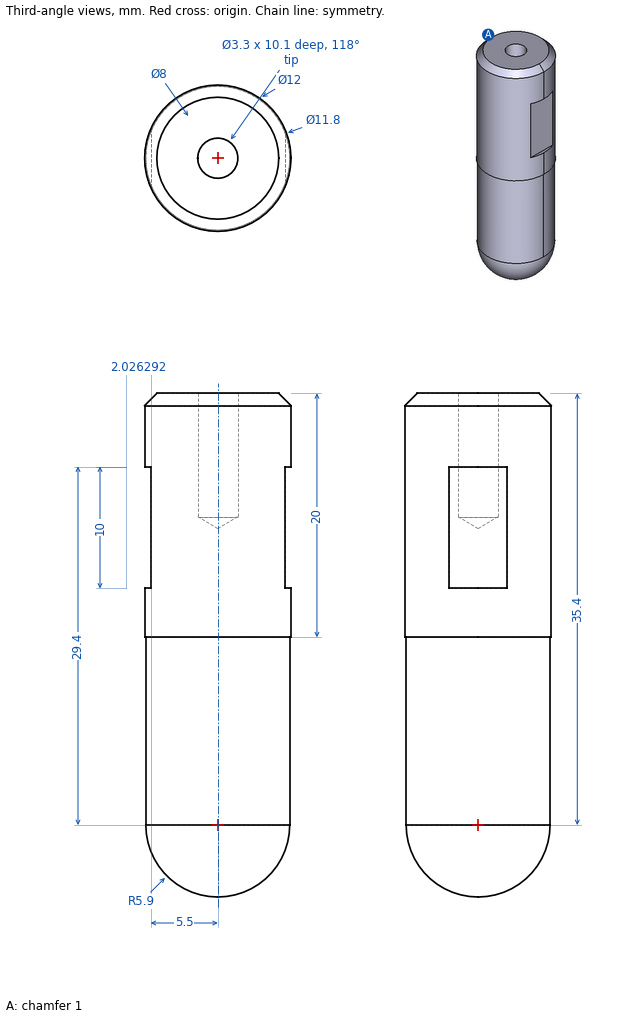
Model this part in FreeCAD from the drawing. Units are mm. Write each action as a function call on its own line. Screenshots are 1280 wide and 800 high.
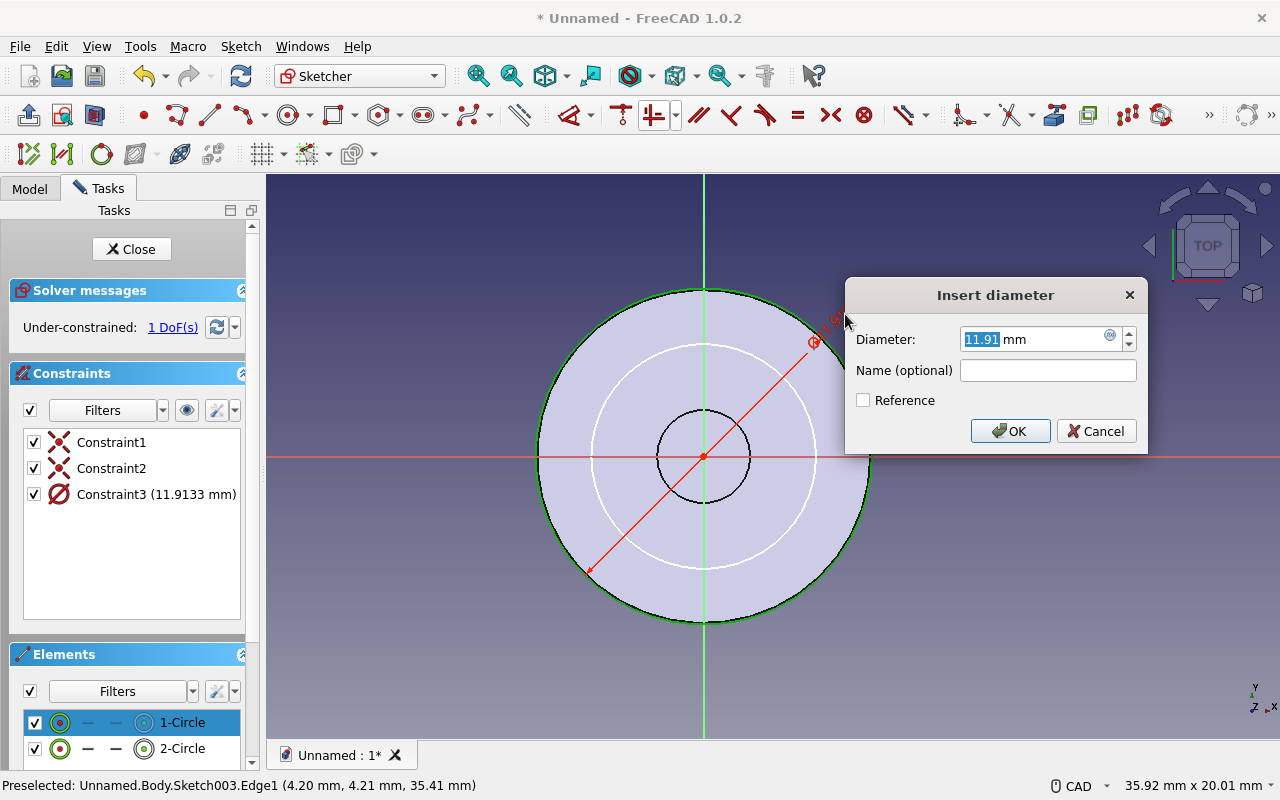
text(12)
key(Return)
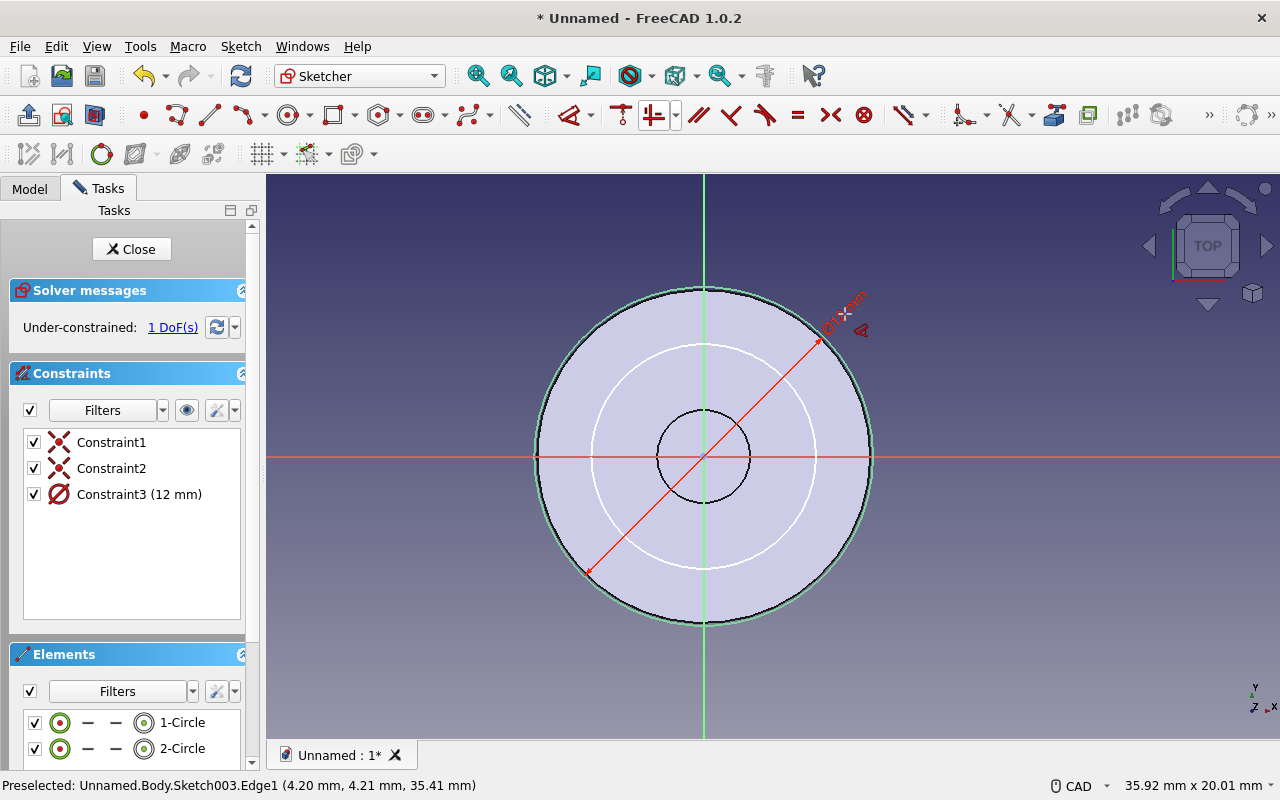
click(783, 377)
click(806, 354)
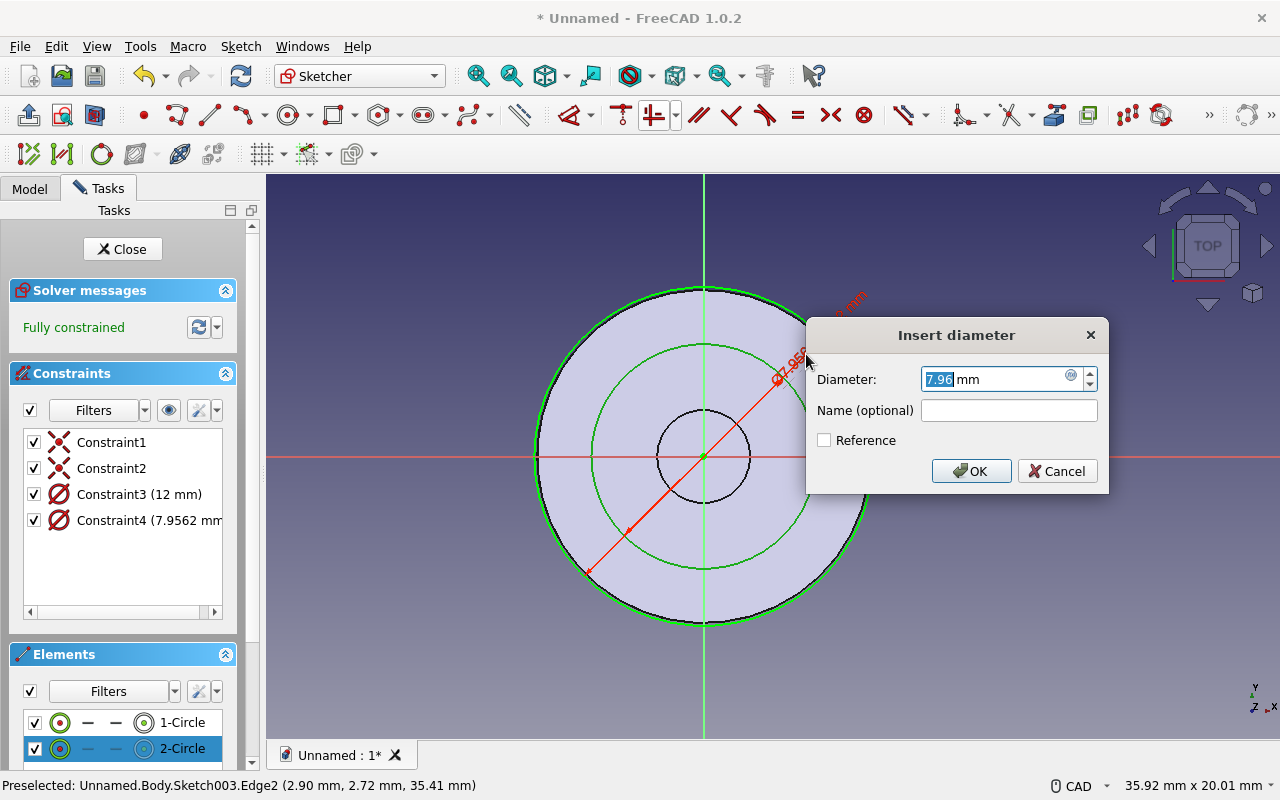
text(8)
key(Return)
key(Escape)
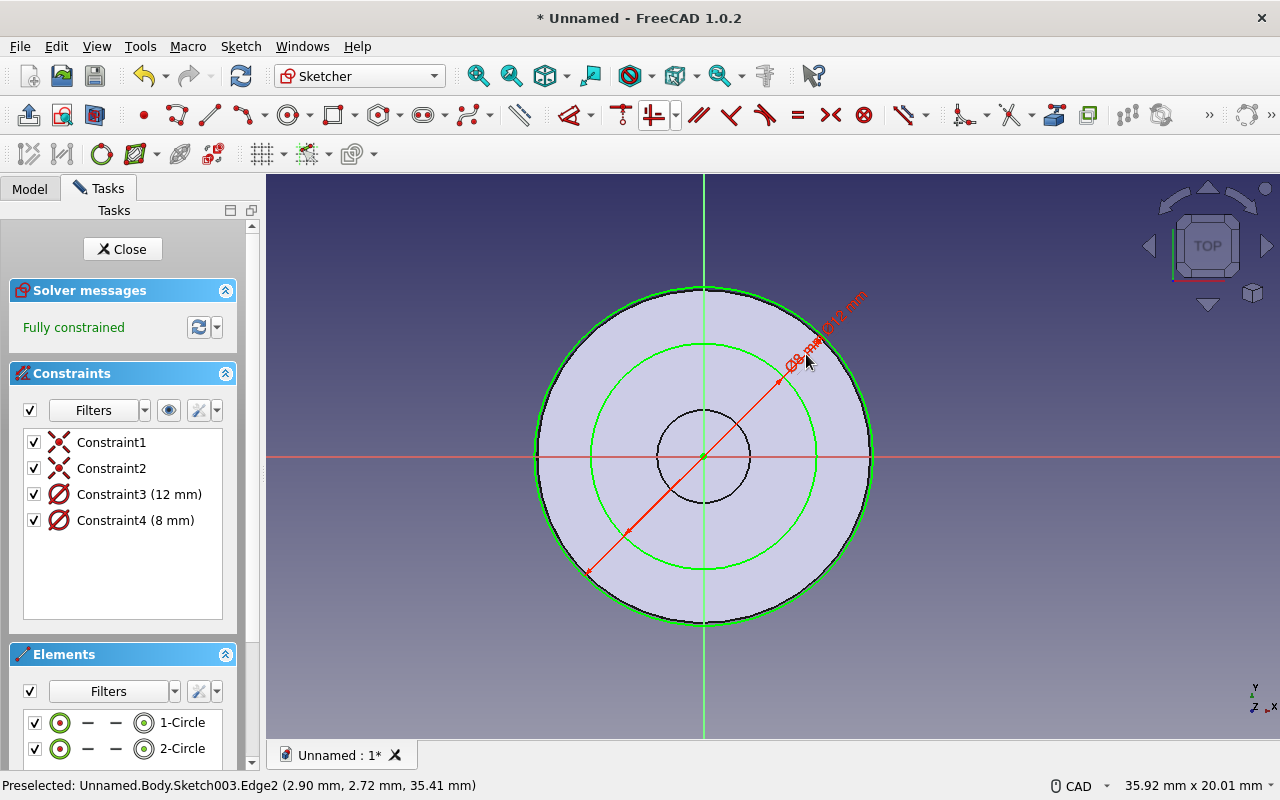
click(123, 249)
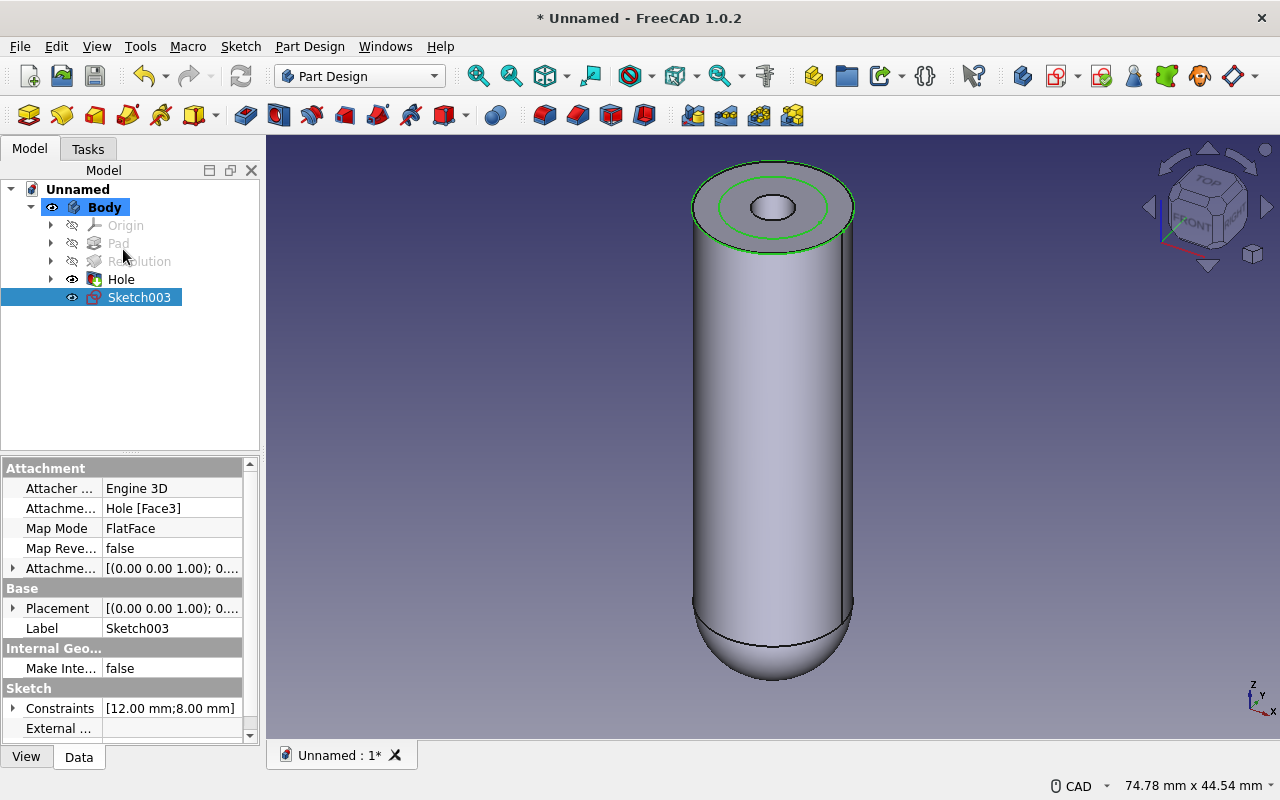
click(29, 116)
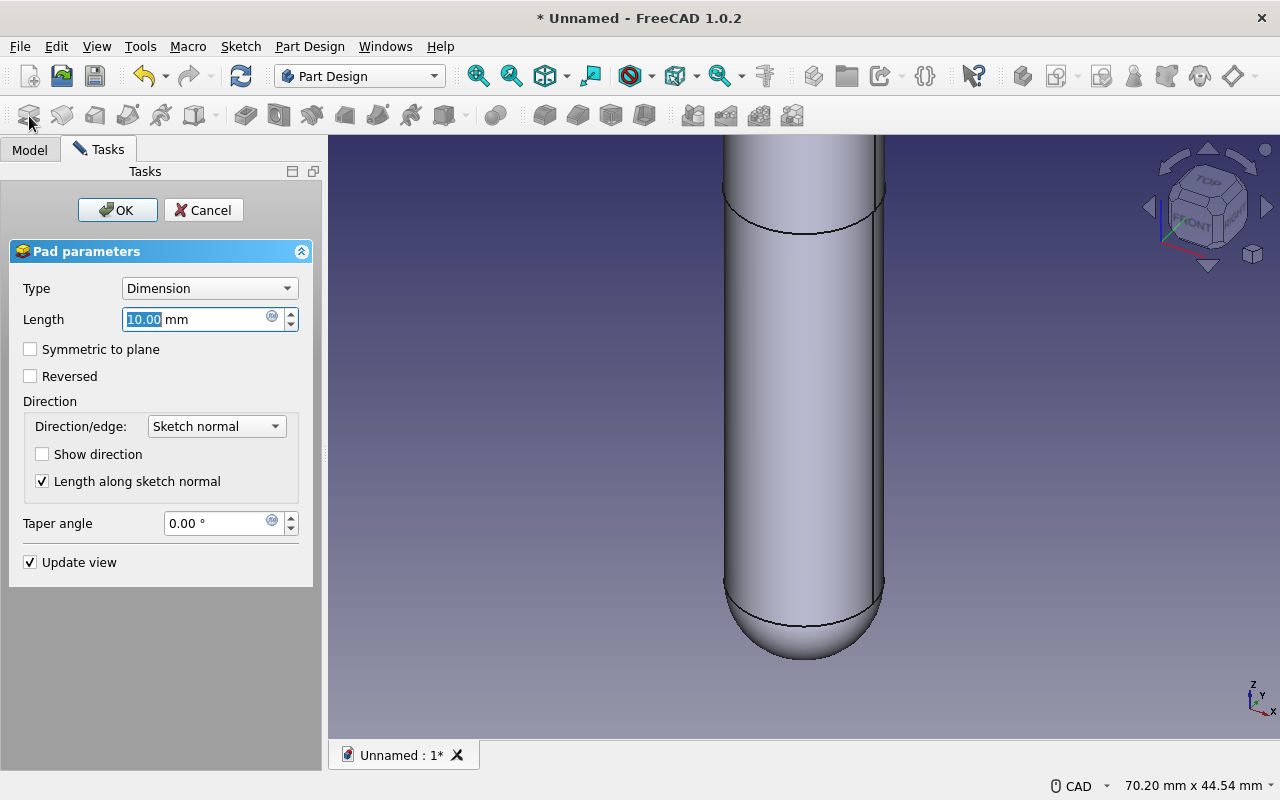
text(20)
key(Tab)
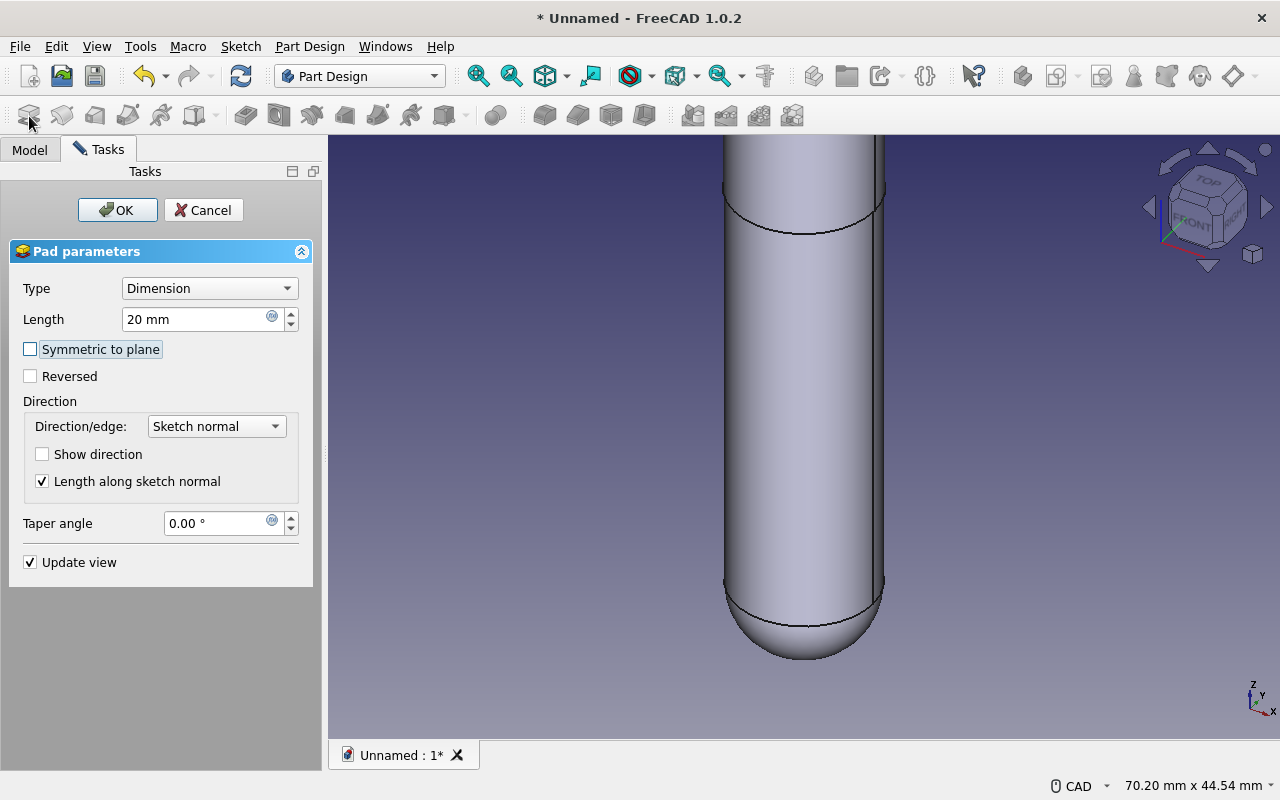
click(31, 376)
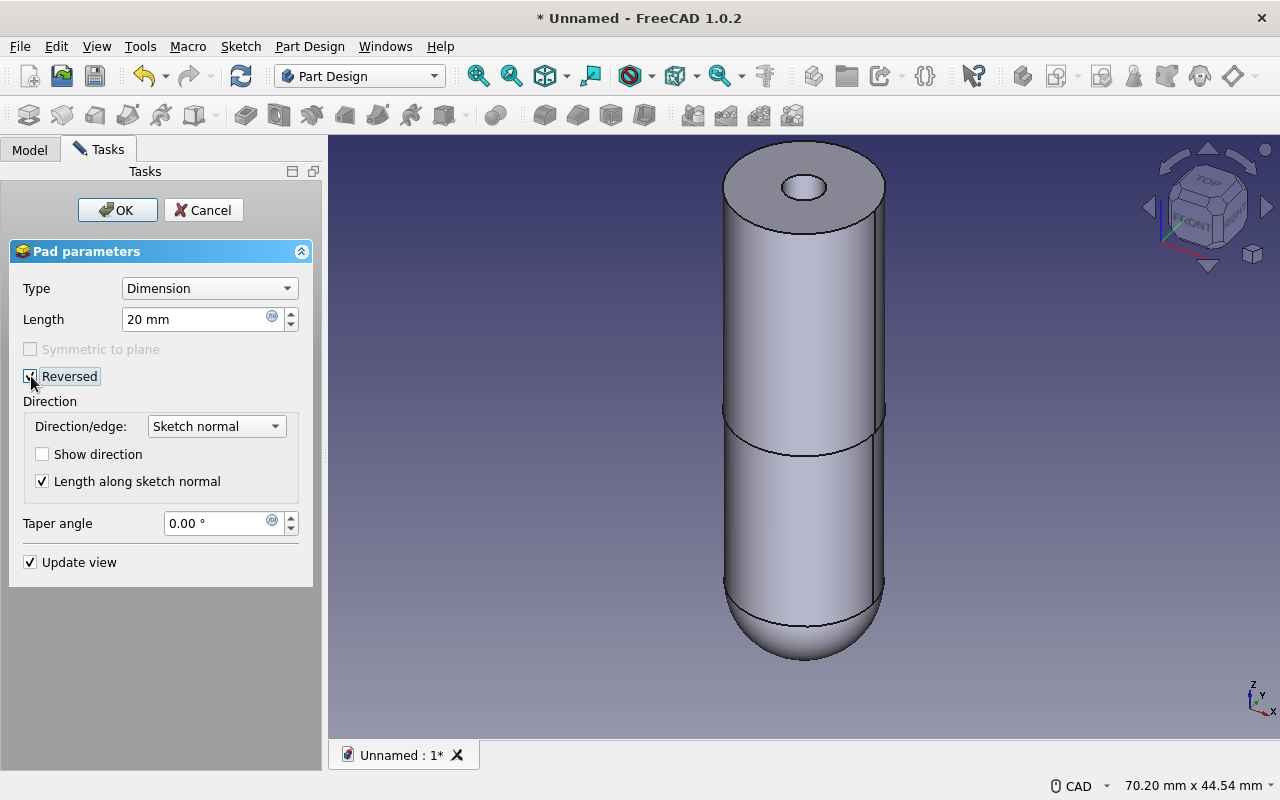
click(118, 210)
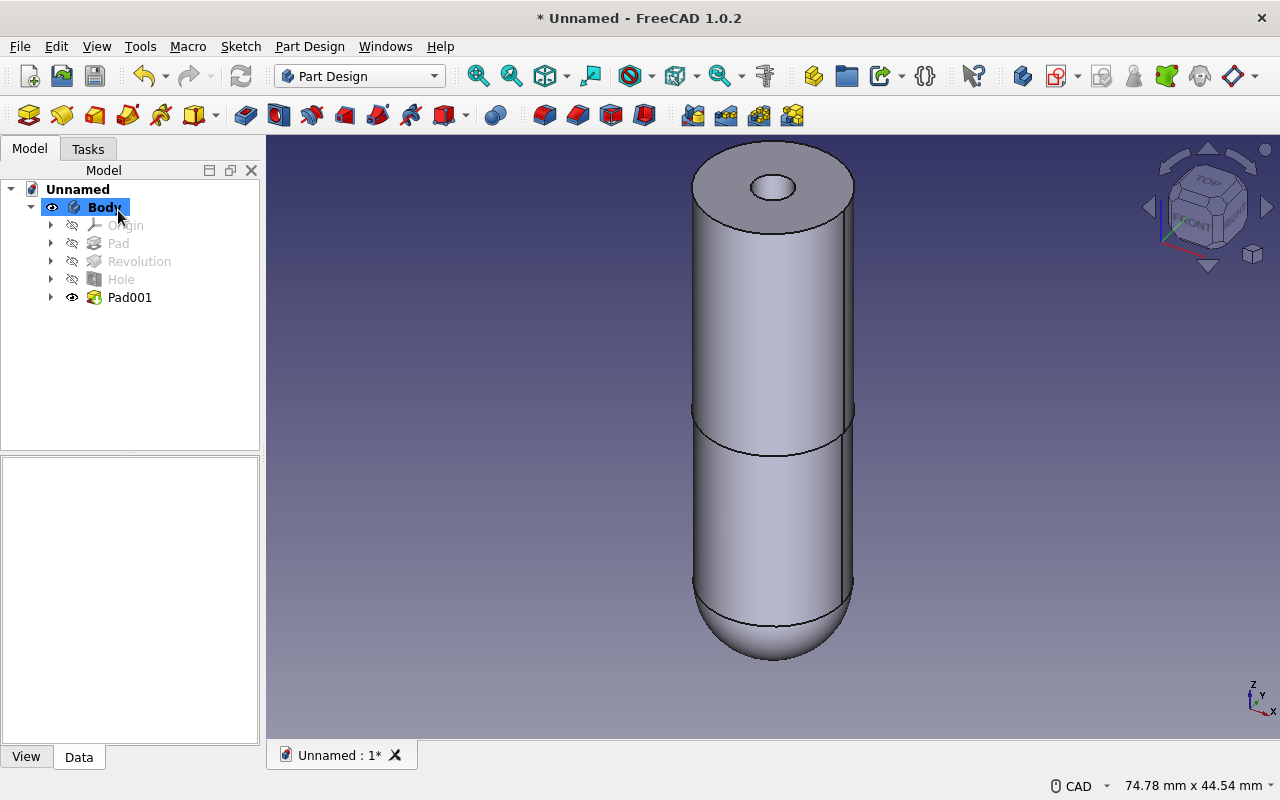
click(479, 76)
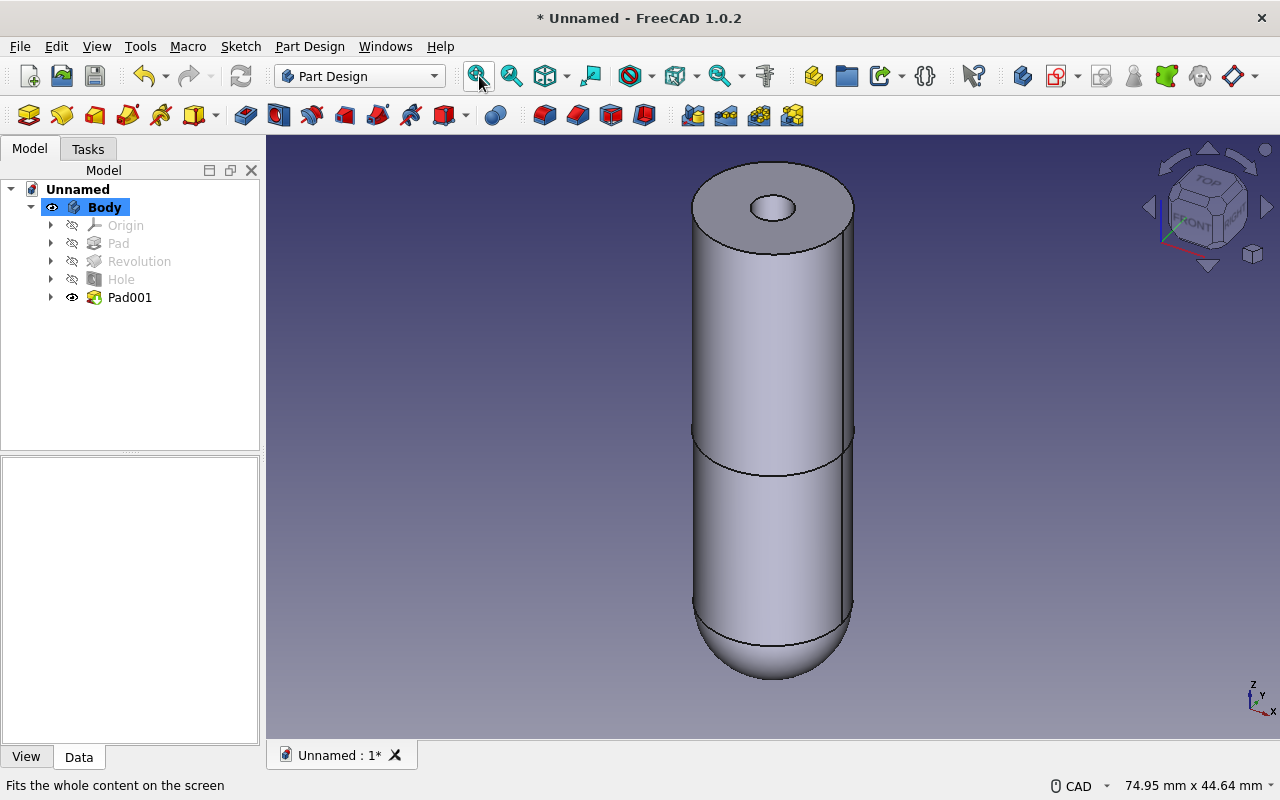
click(692, 212)